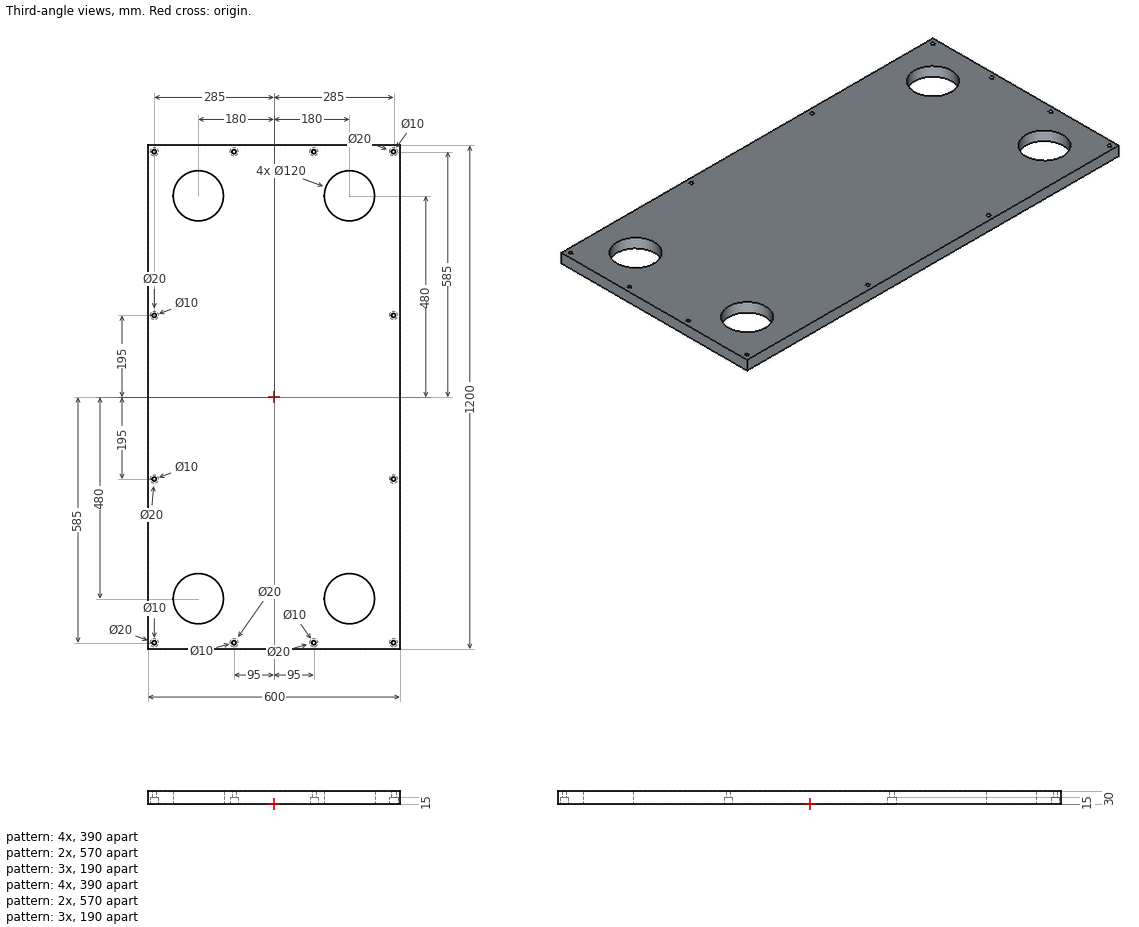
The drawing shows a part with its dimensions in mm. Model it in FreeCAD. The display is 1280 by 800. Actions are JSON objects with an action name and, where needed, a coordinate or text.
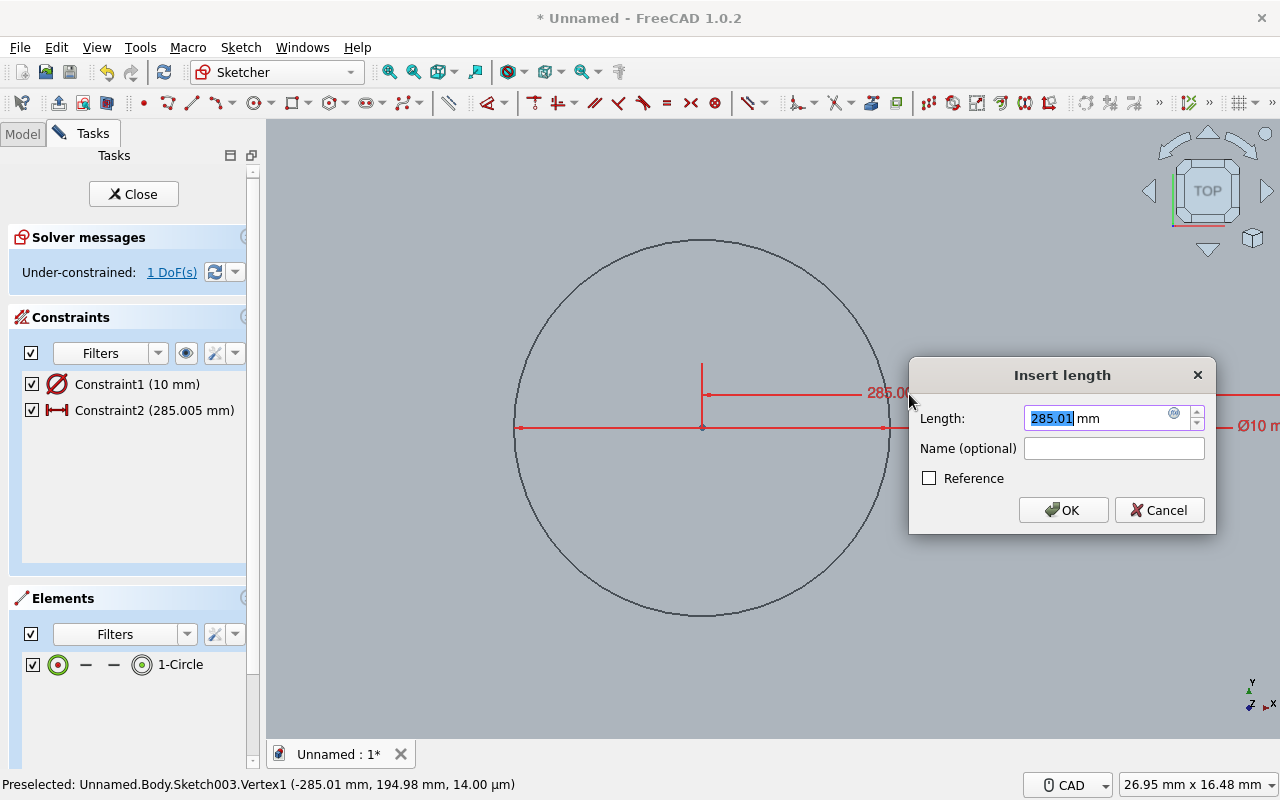
{"action": "type", "text": "285"}
{"action": "key", "text": "Return"}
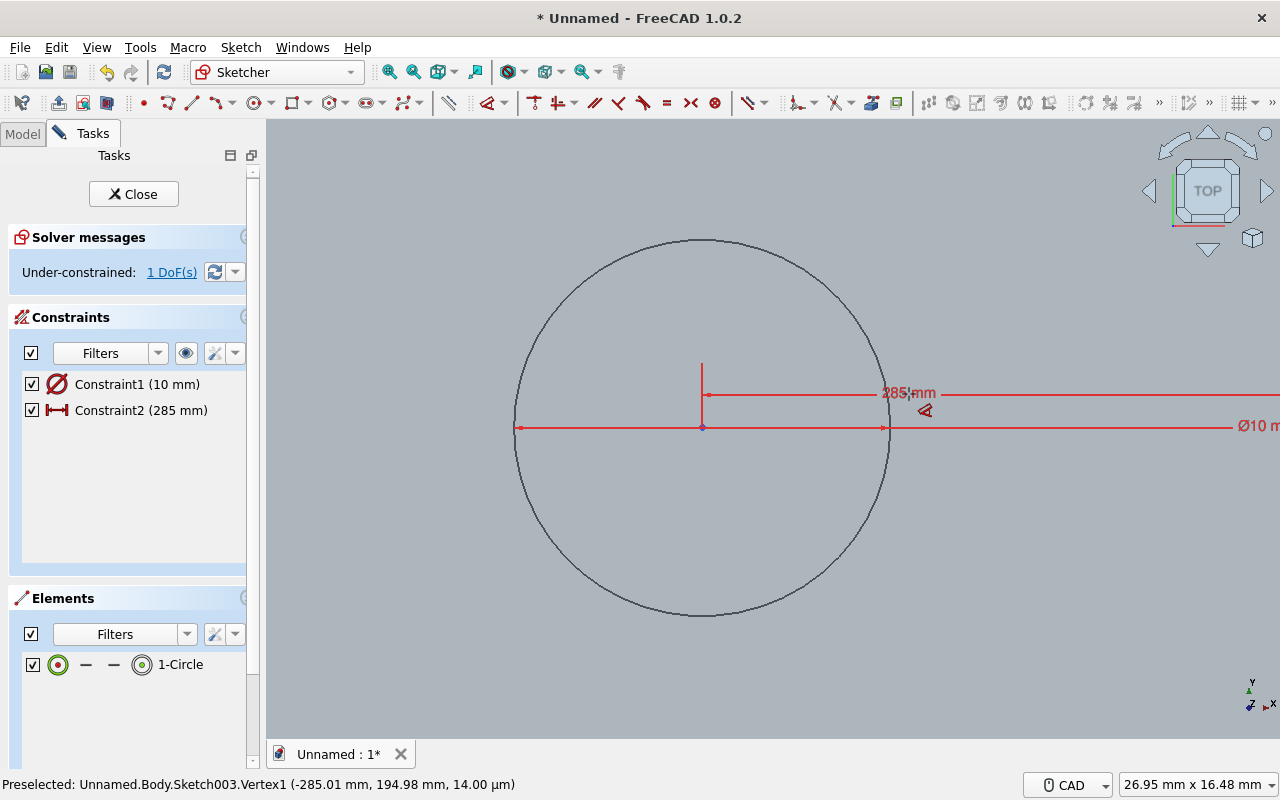
{"action": "left_click", "coordinate": [702, 428]}
{"action": "left_click", "coordinate": [668, 569]}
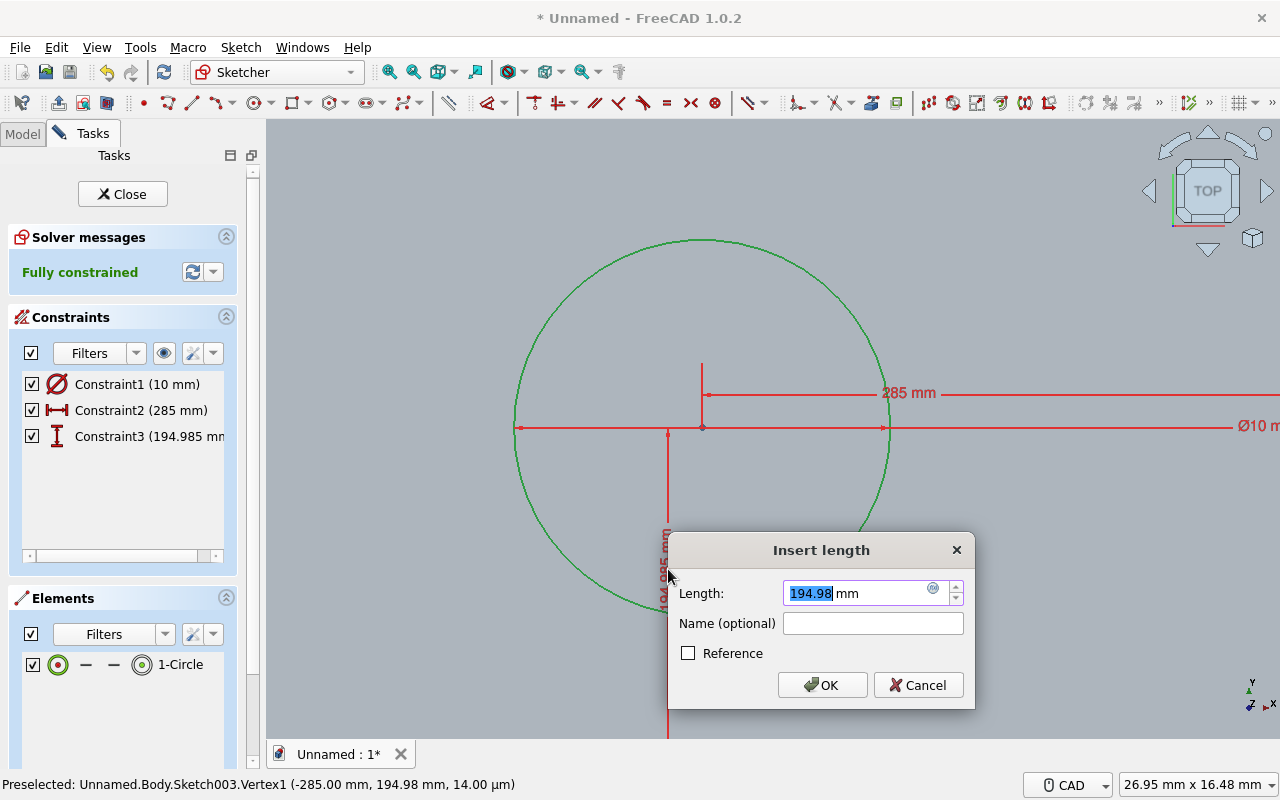
{"action": "type", "text": "195"}
{"action": "key", "text": "Return"}
{"action": "key", "text": "Escape"}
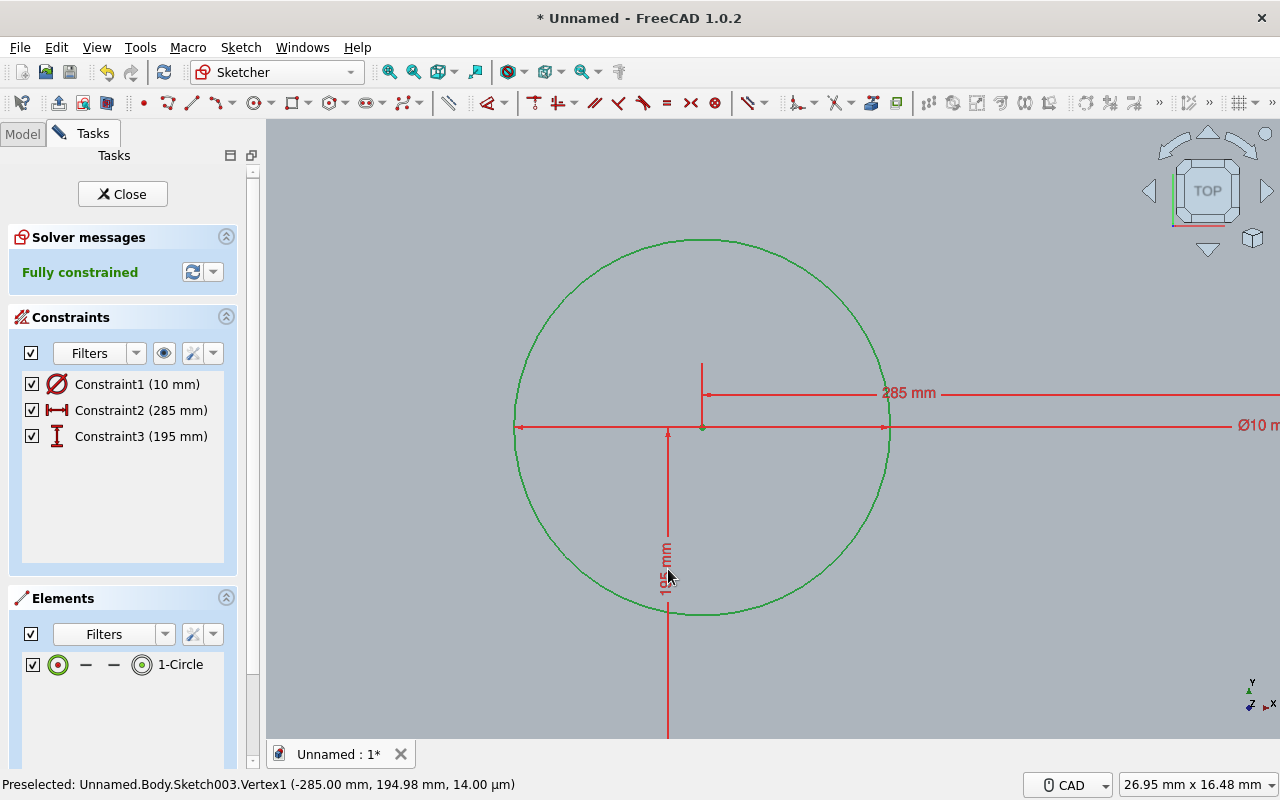
{"action": "left_click", "coordinate": [123, 194]}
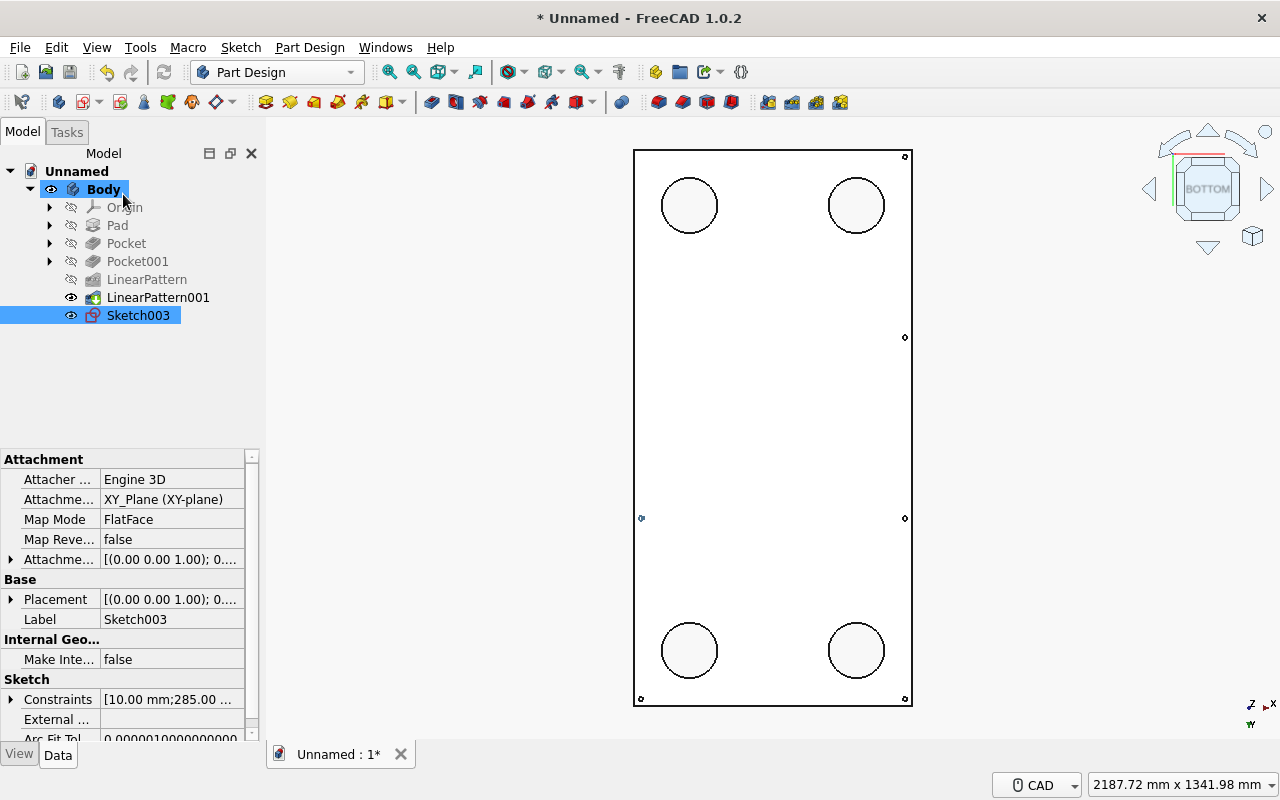
{"action": "left_click", "coordinate": [432, 102]}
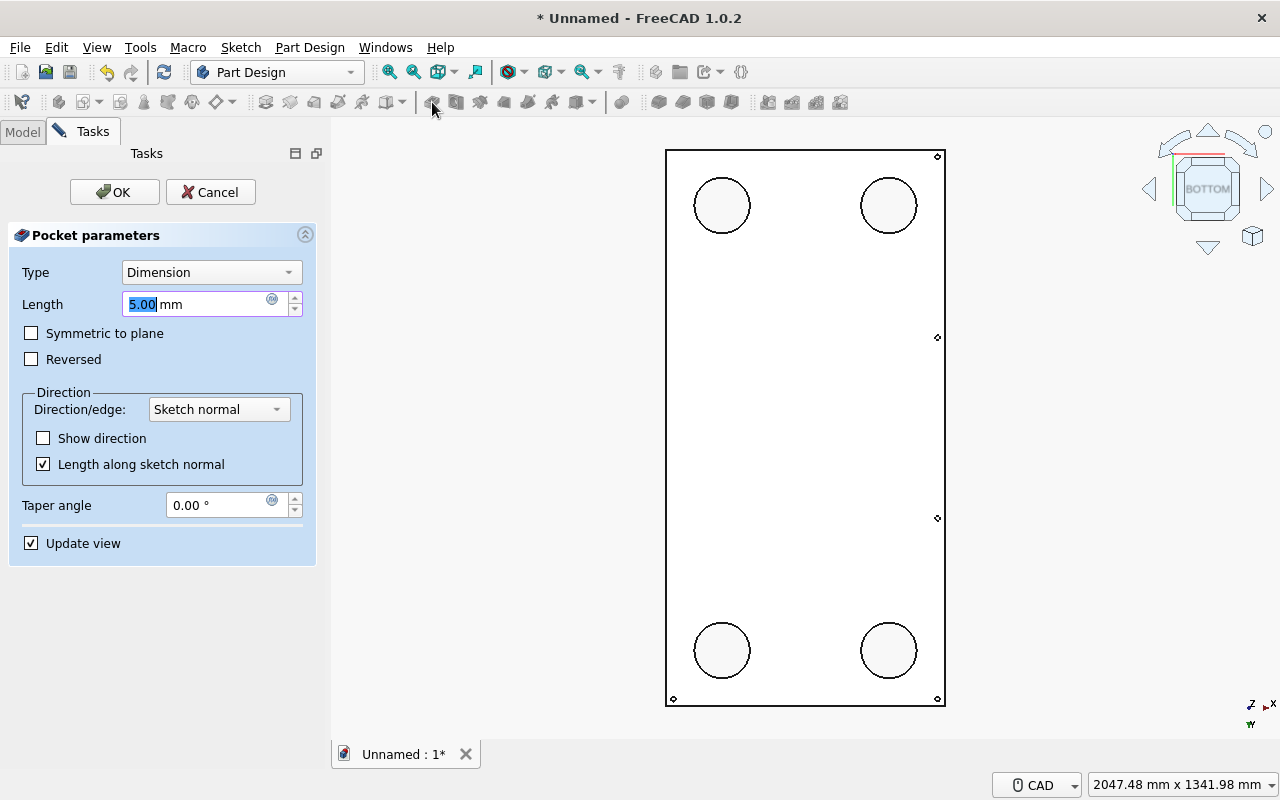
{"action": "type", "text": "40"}
{"action": "key", "text": "Tab"}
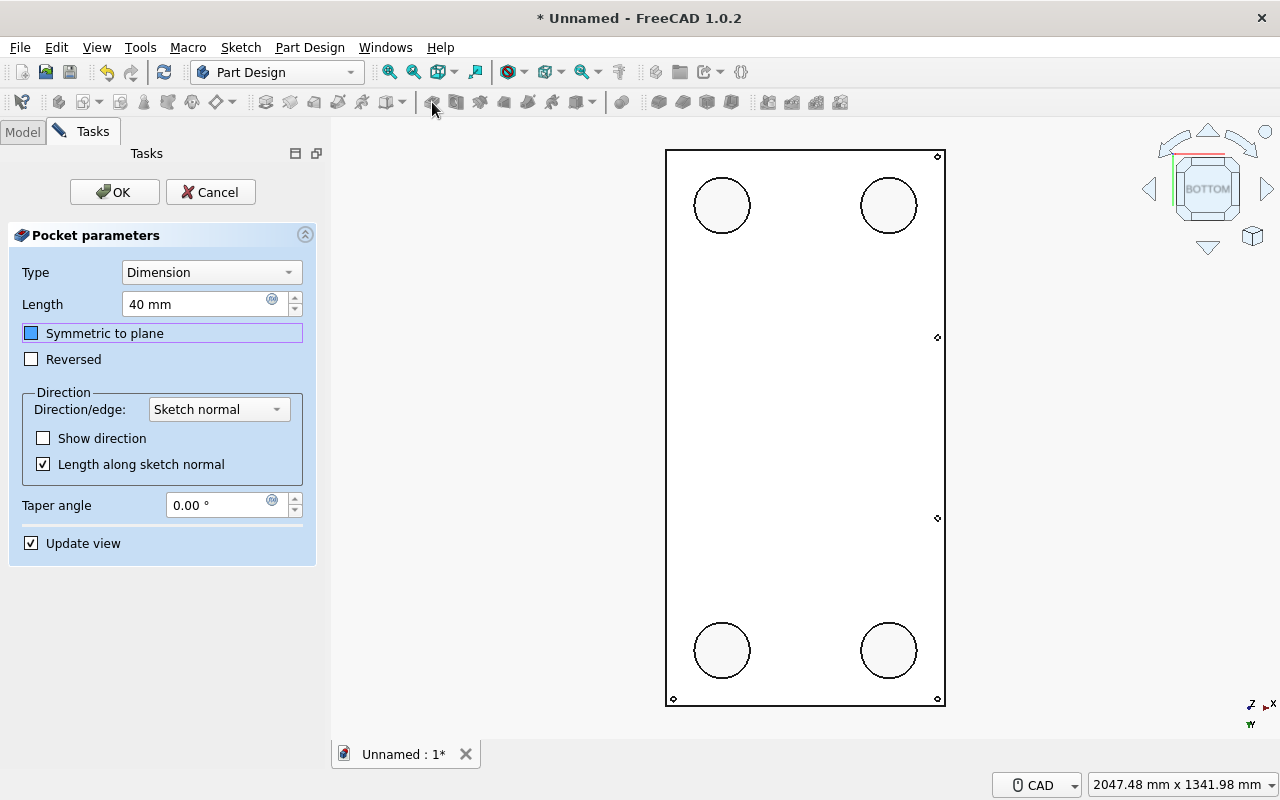
{"action": "left_click", "coordinate": [30, 359]}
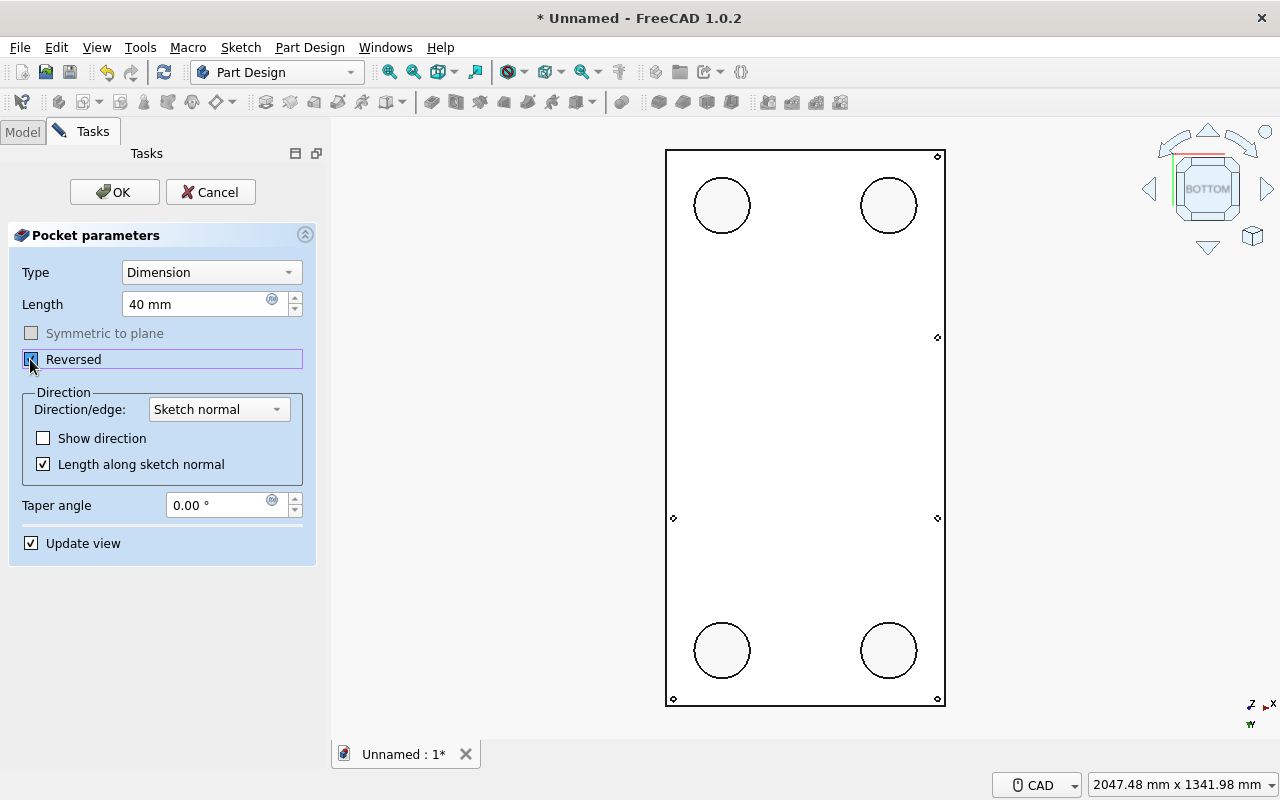
{"action": "left_click", "coordinate": [115, 192]}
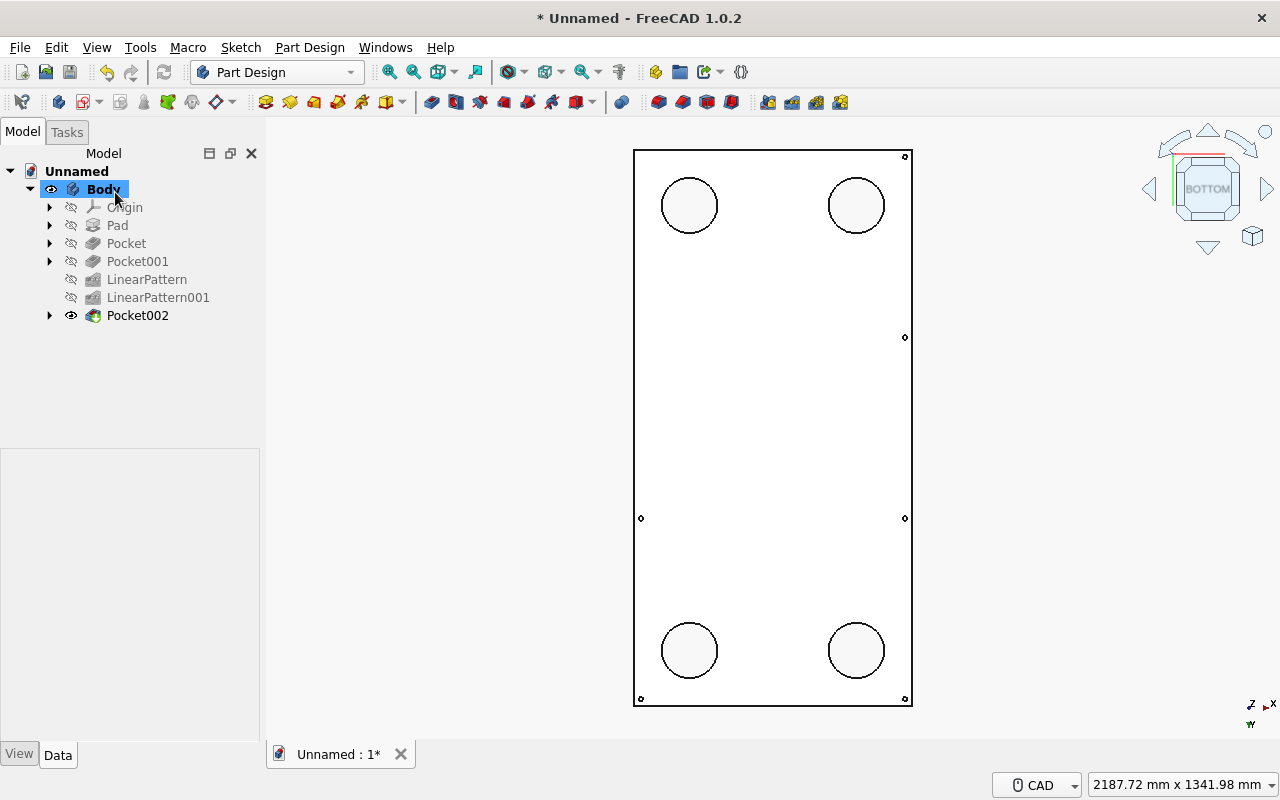
{"action": "left_click", "coordinate": [84, 102]}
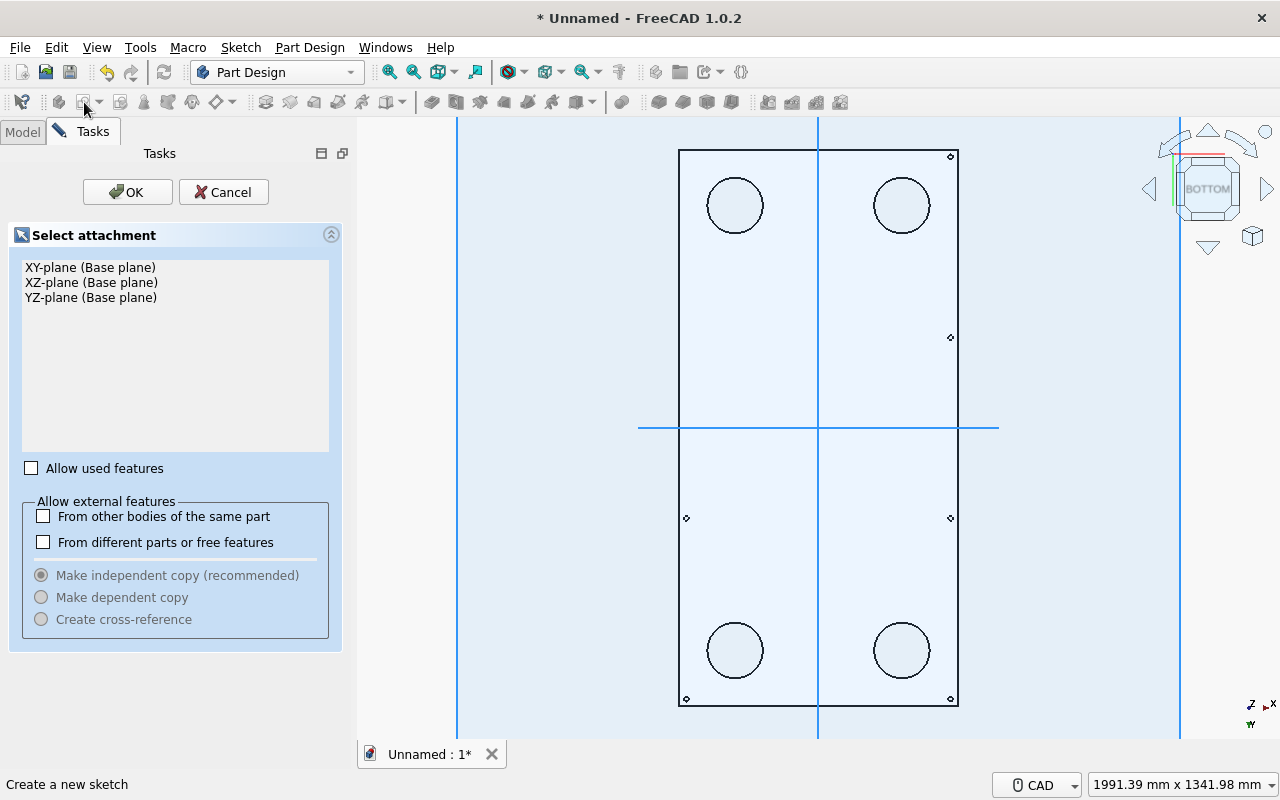
{"action": "left_click", "coordinate": [82, 268]}